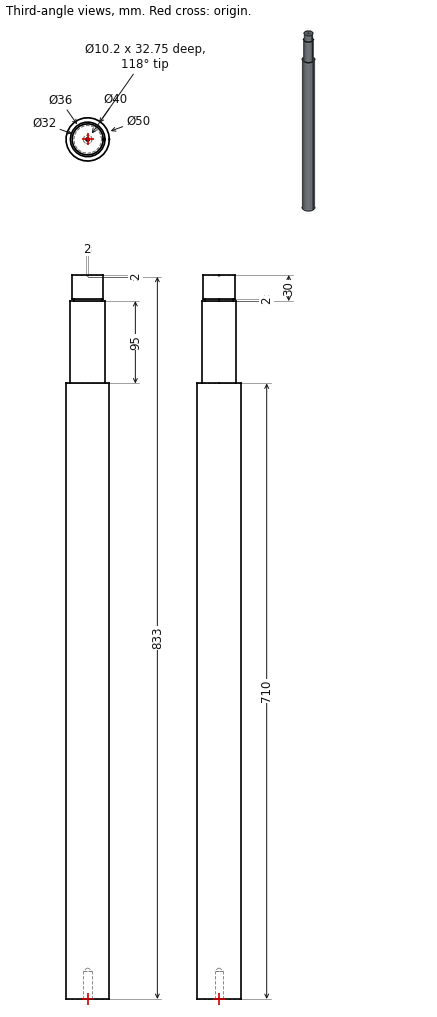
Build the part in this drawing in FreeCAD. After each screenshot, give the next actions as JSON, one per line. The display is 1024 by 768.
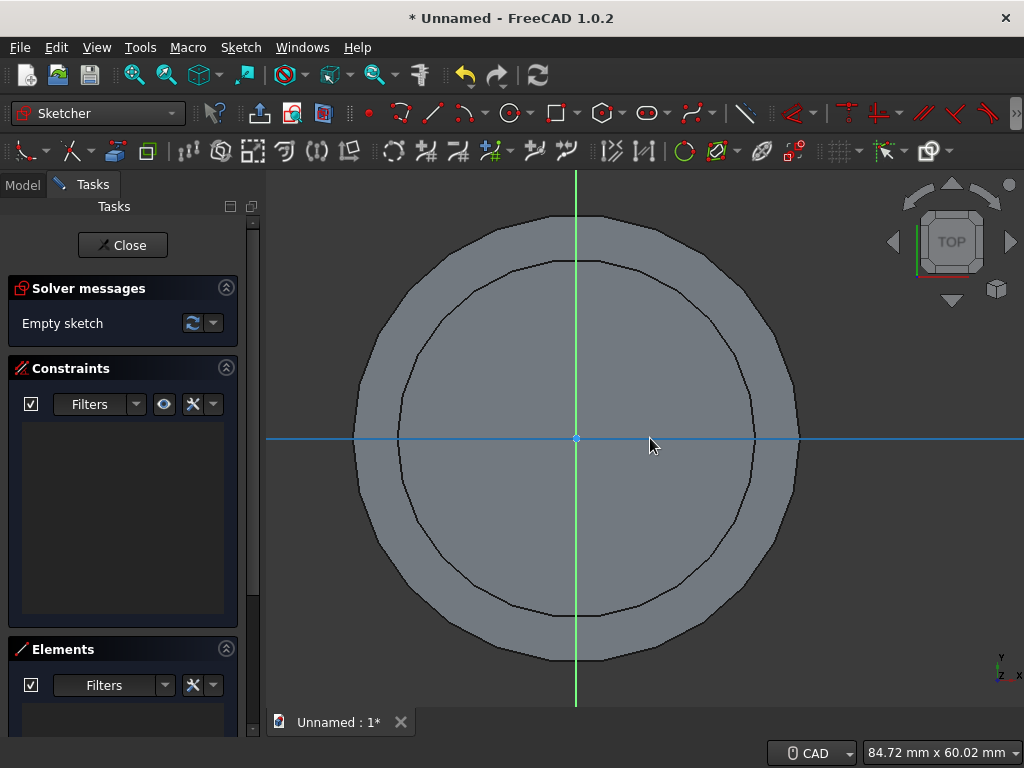
{"action": "left_click", "coordinate": [510, 114]}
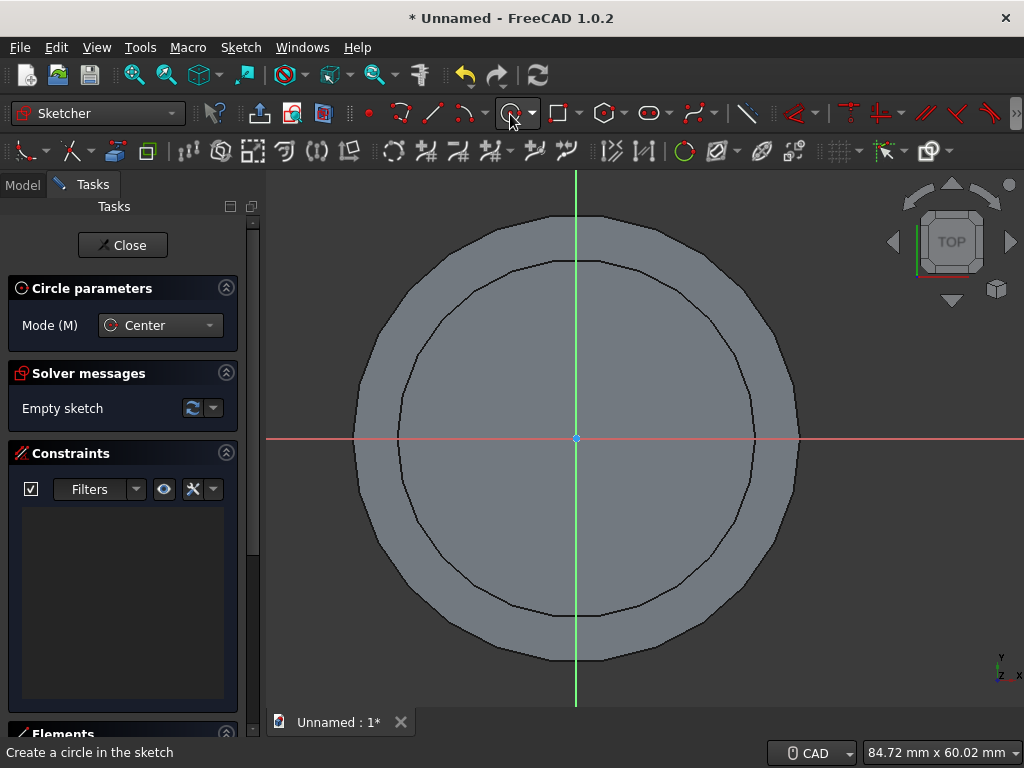
{"action": "left_click", "coordinate": [576, 438]}
{"action": "mouse_move", "coordinate": [690, 325]}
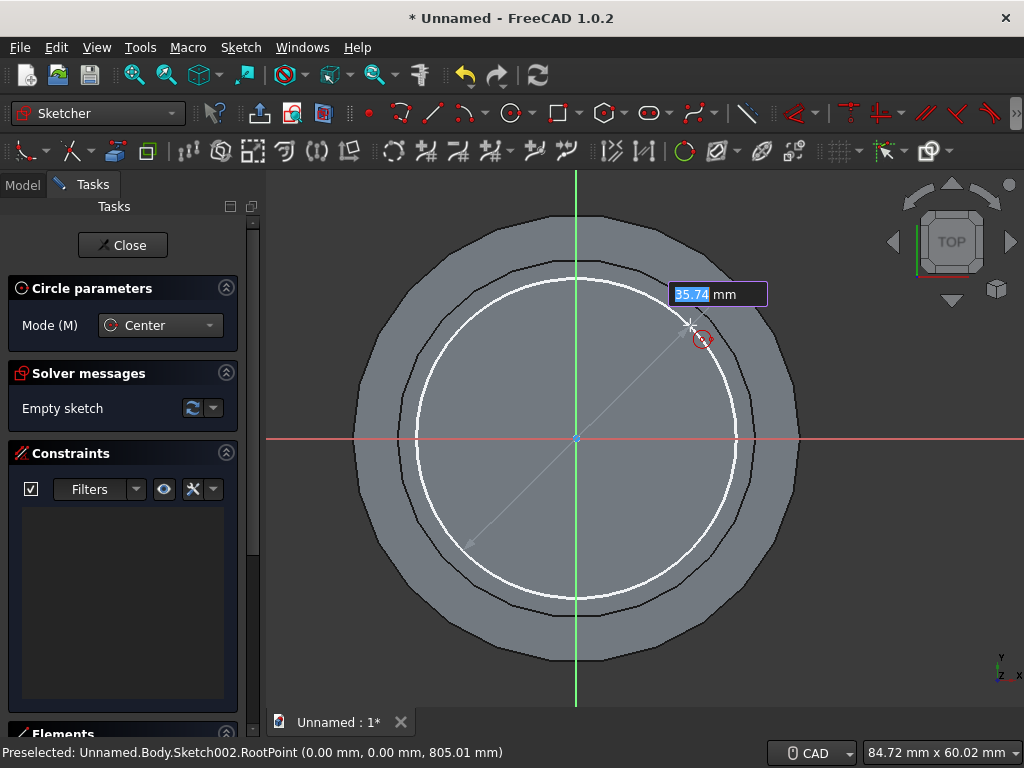
{"action": "type", "text": "36"}
{"action": "key", "text": "Return"}
{"action": "key", "text": "Escape"}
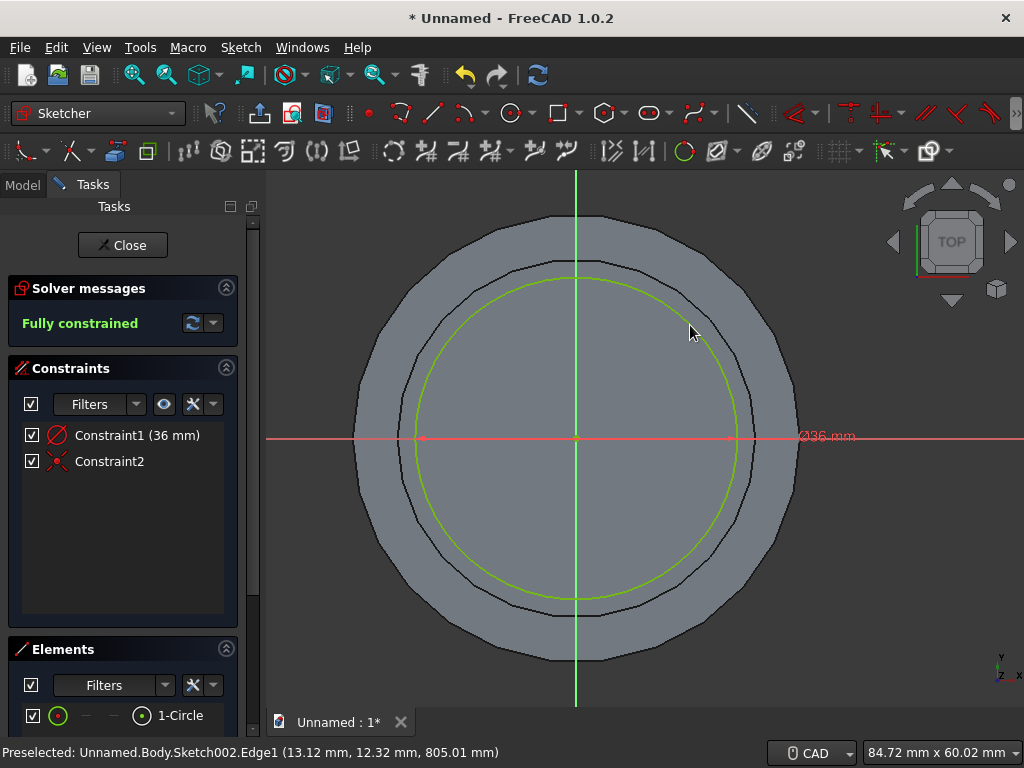
{"action": "left_click", "coordinate": [123, 245]}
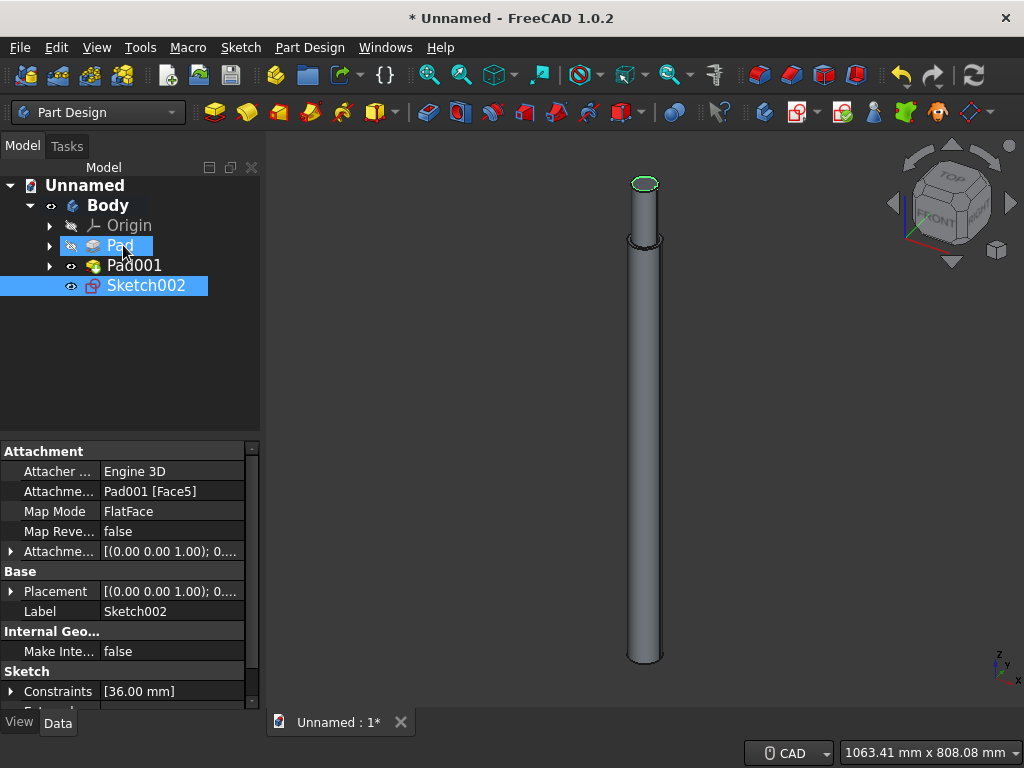
{"action": "left_click", "coordinate": [216, 112]}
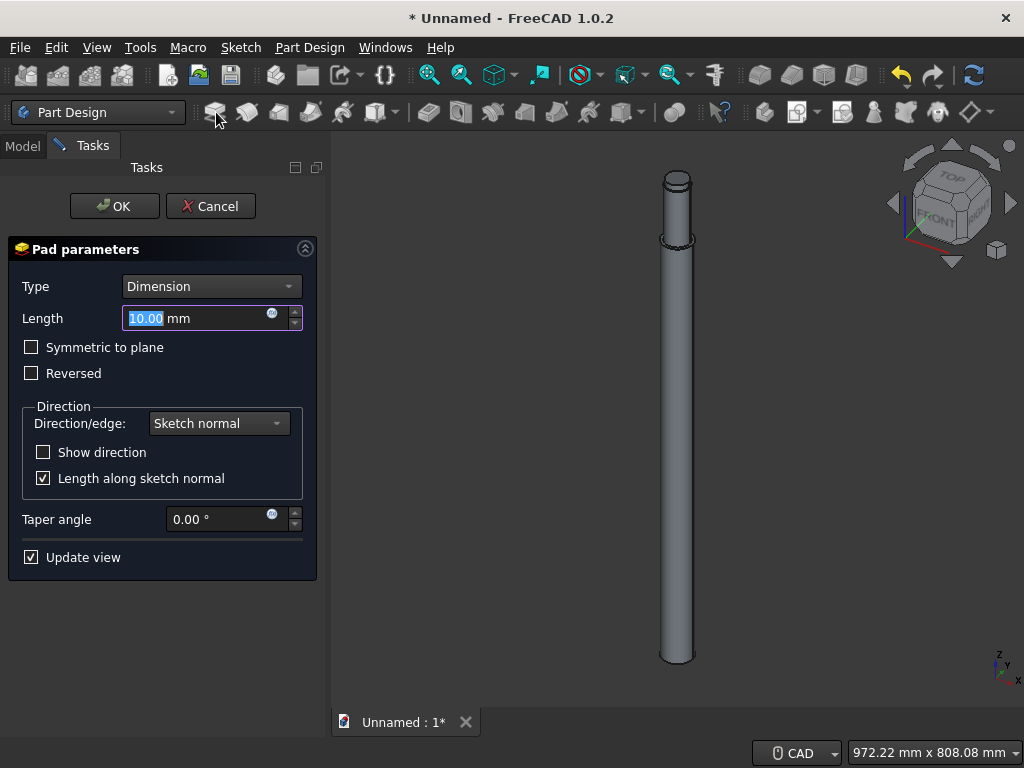
{"action": "type", "text": "30"}
{"action": "key", "text": "Tab"}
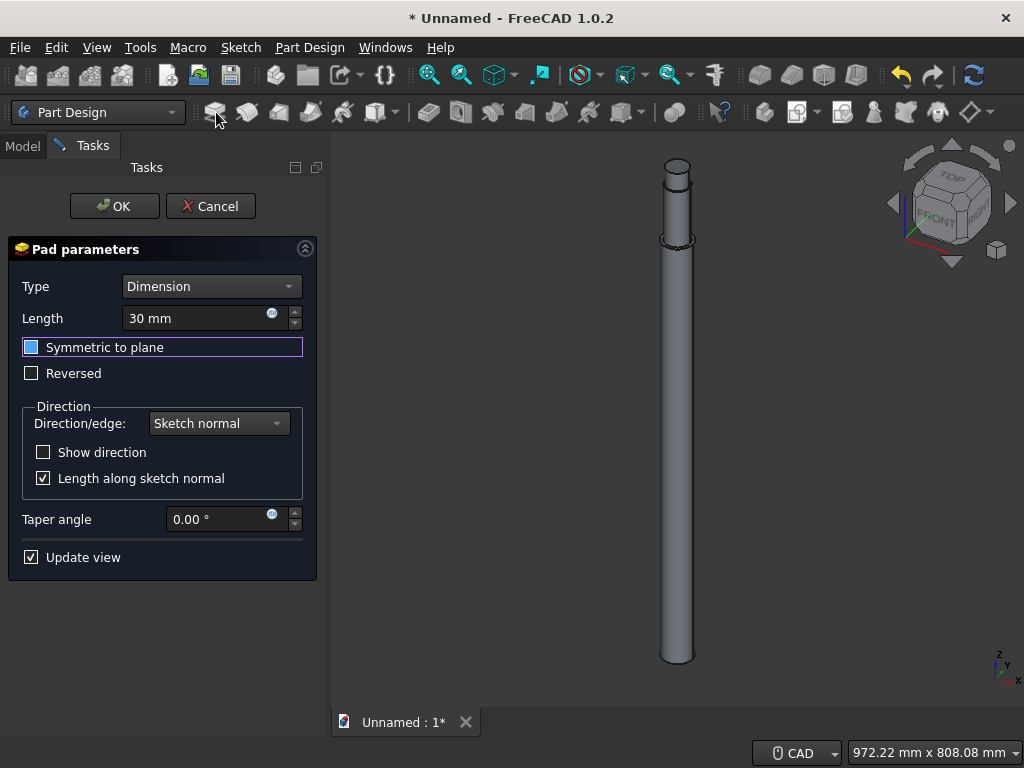
{"action": "left_click", "coordinate": [115, 206]}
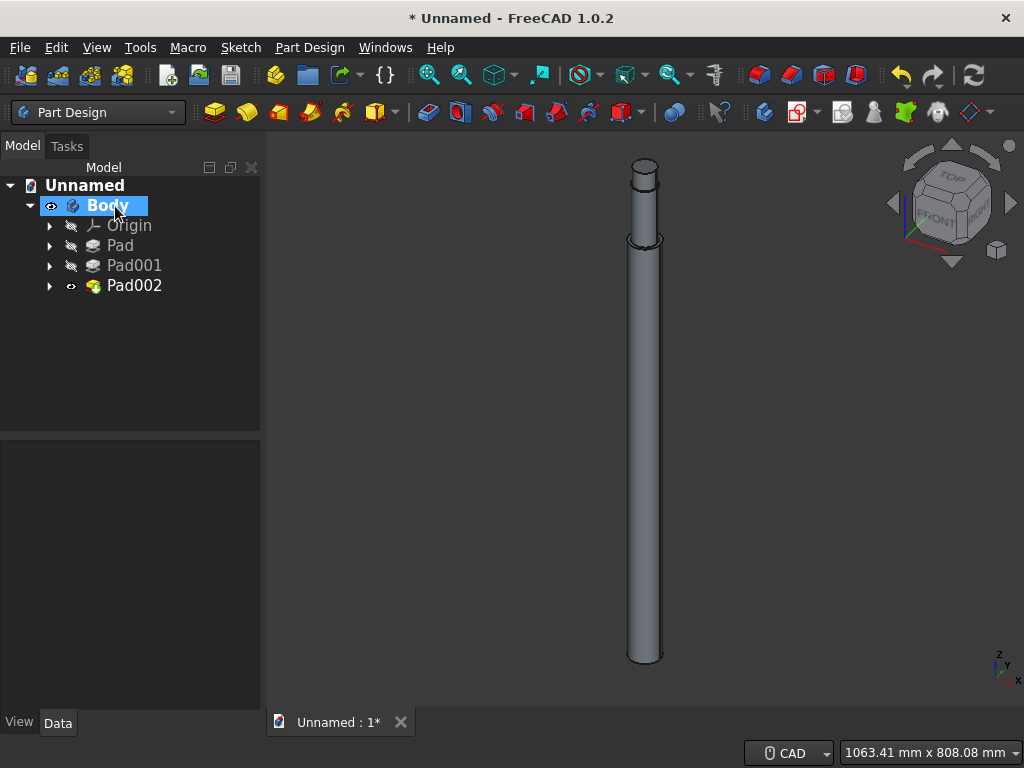
{"action": "left_click", "coordinate": [798, 112]}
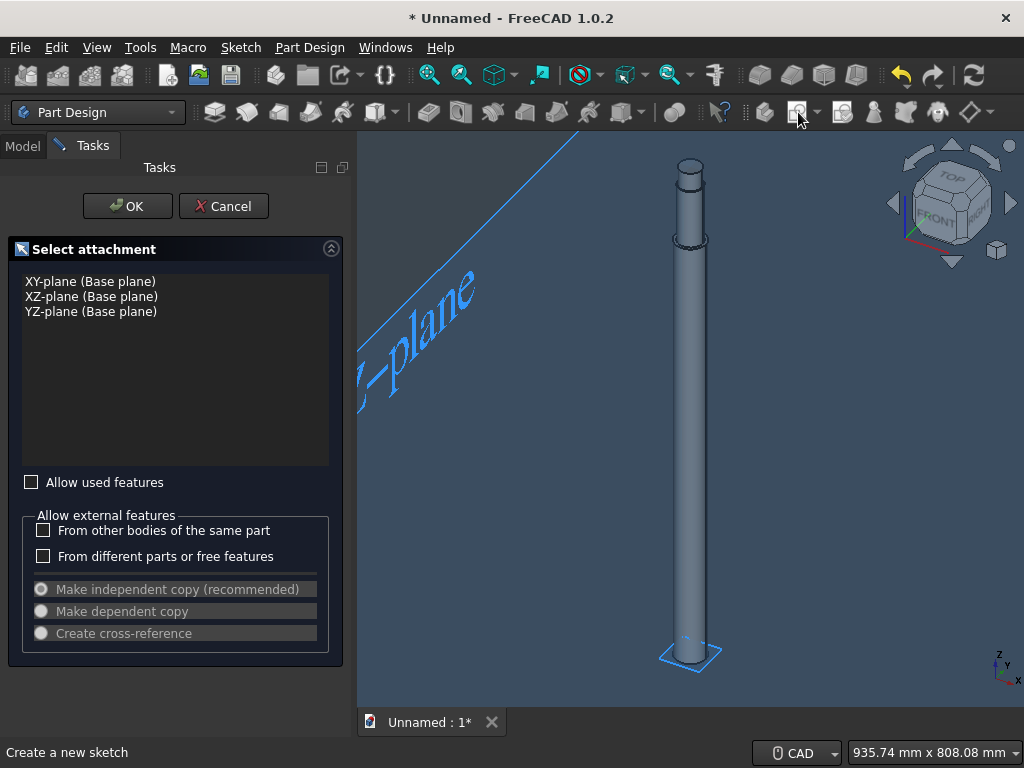
{"action": "left_click", "coordinate": [82, 282]}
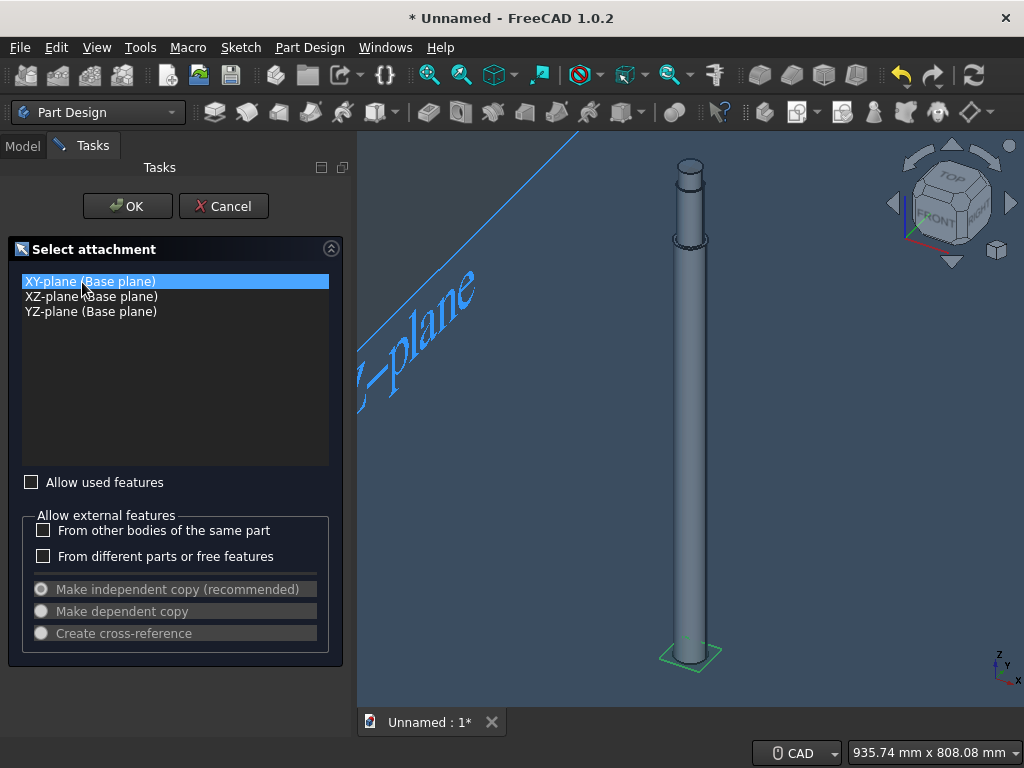
{"action": "left_click", "coordinate": [128, 206]}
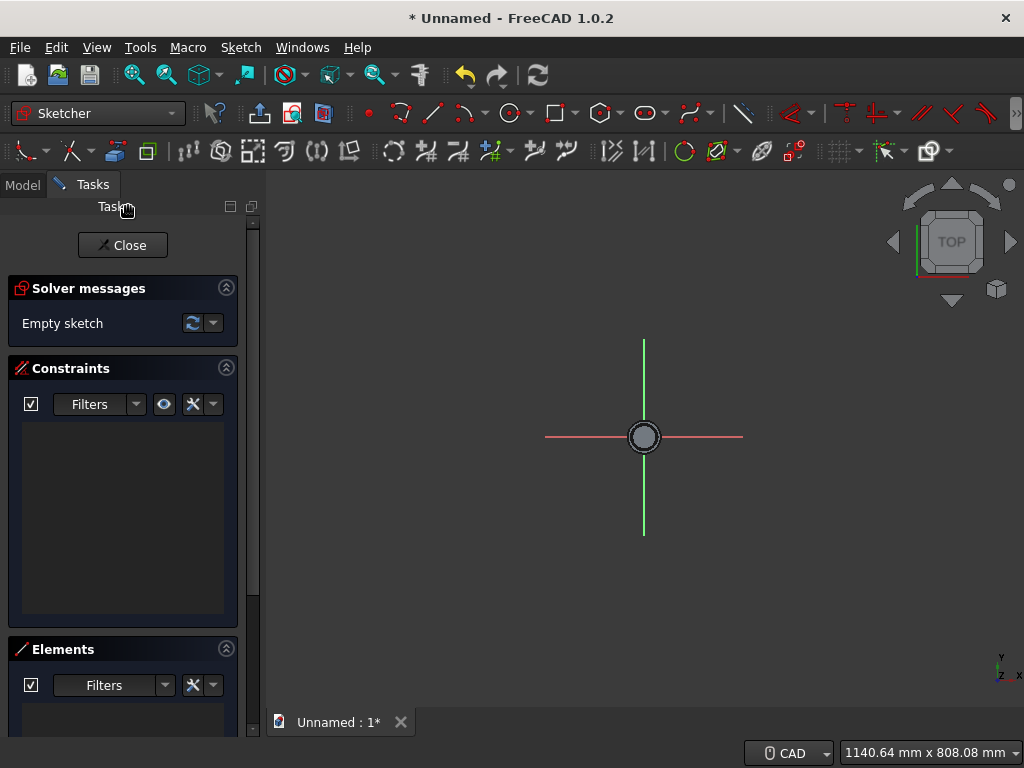
{"action": "left_click", "coordinate": [324, 114]}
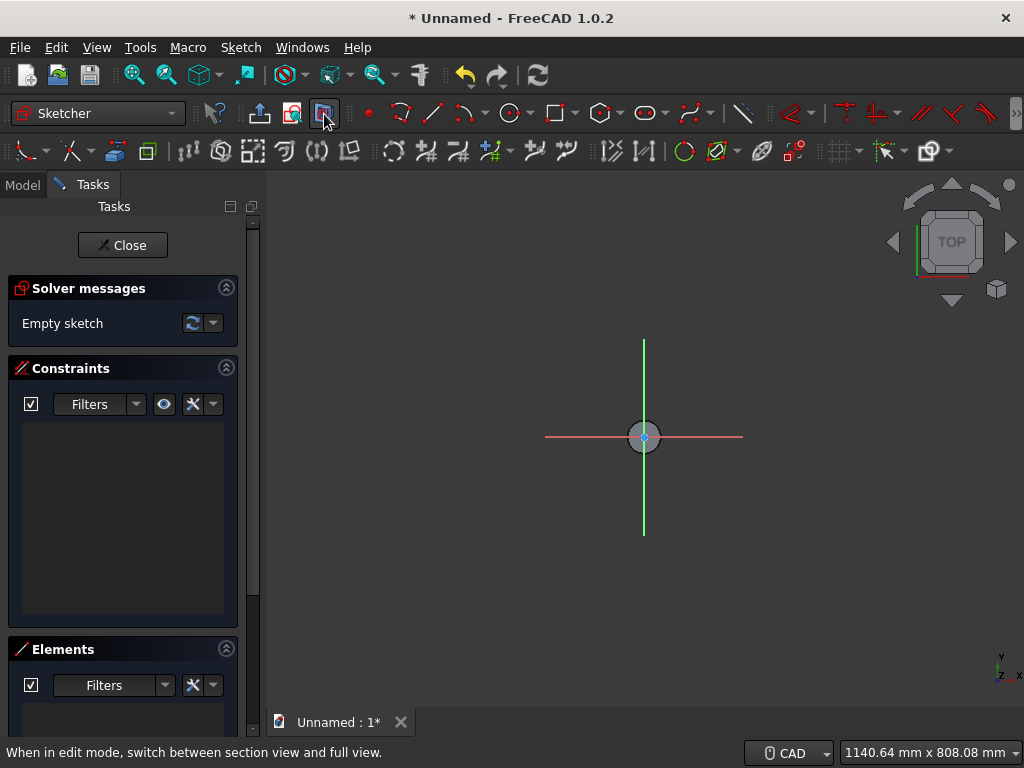
{"action": "scroll", "coordinate": [648, 437], "scroll_direction": "up", "scroll_amount": 15}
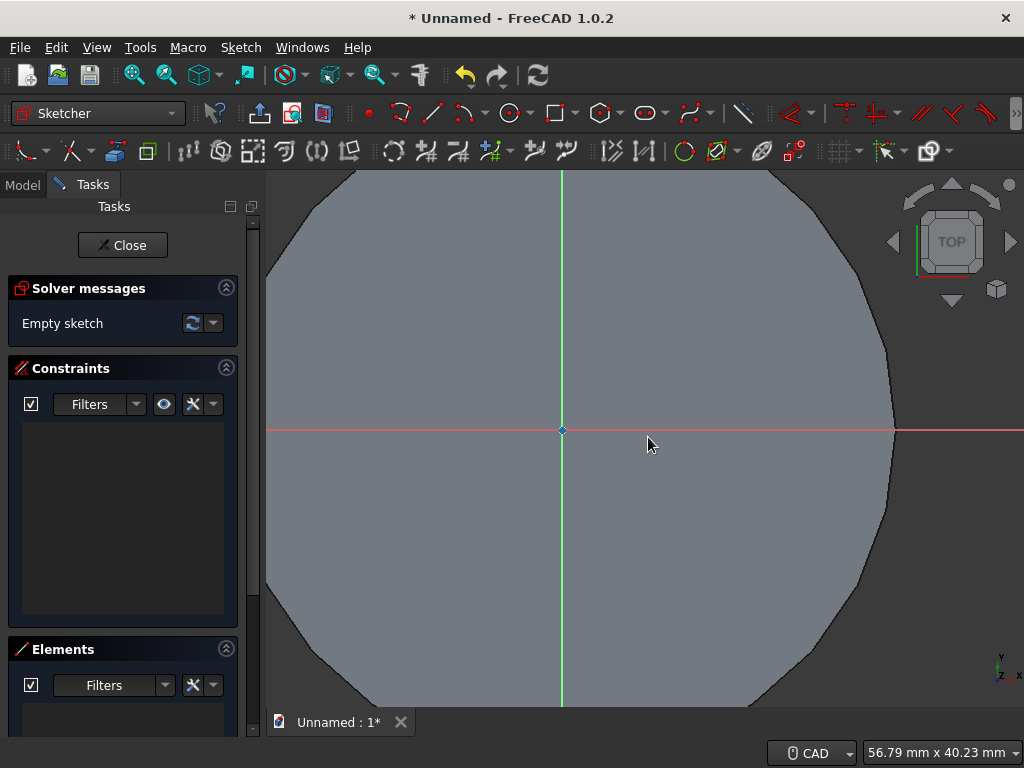
{"action": "scroll", "coordinate": [554, 425], "scroll_direction": "up", "scroll_amount": 5}